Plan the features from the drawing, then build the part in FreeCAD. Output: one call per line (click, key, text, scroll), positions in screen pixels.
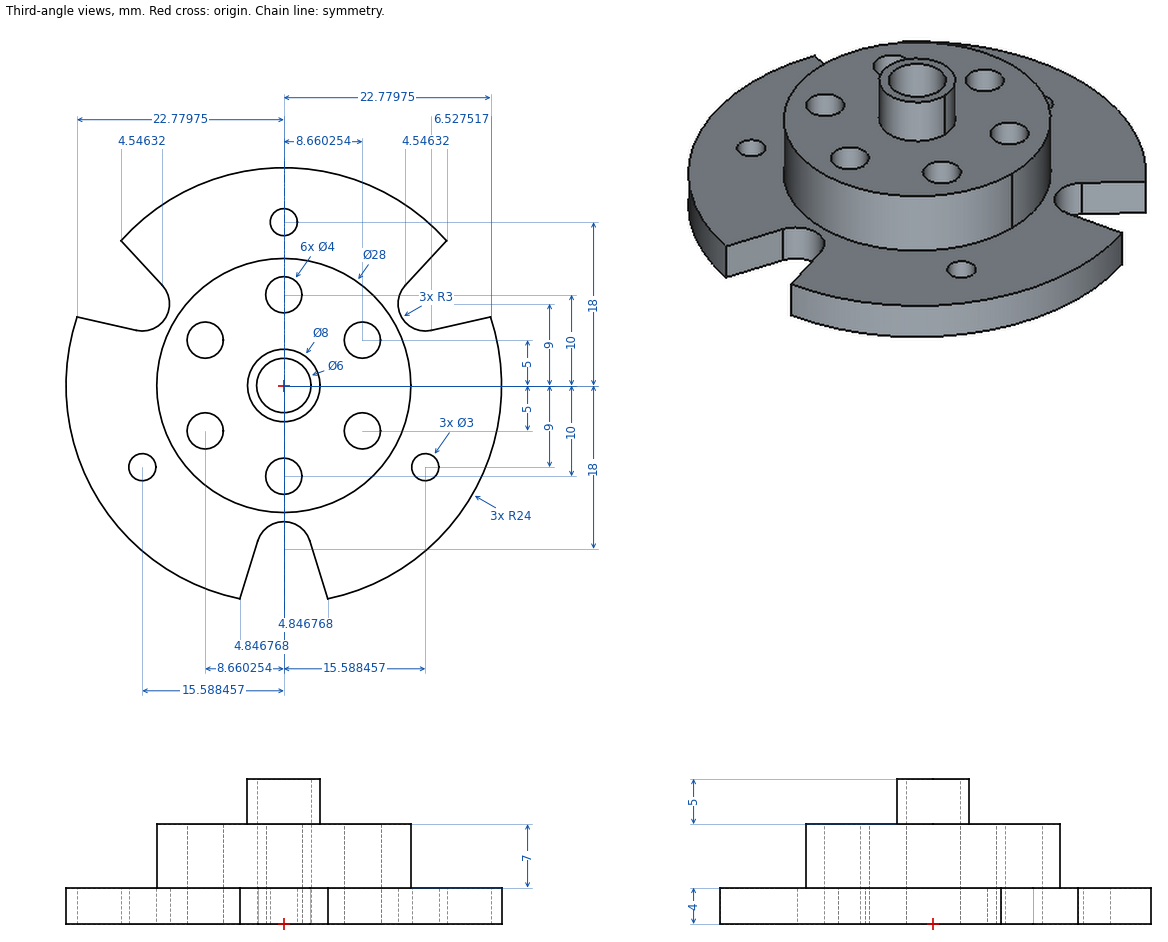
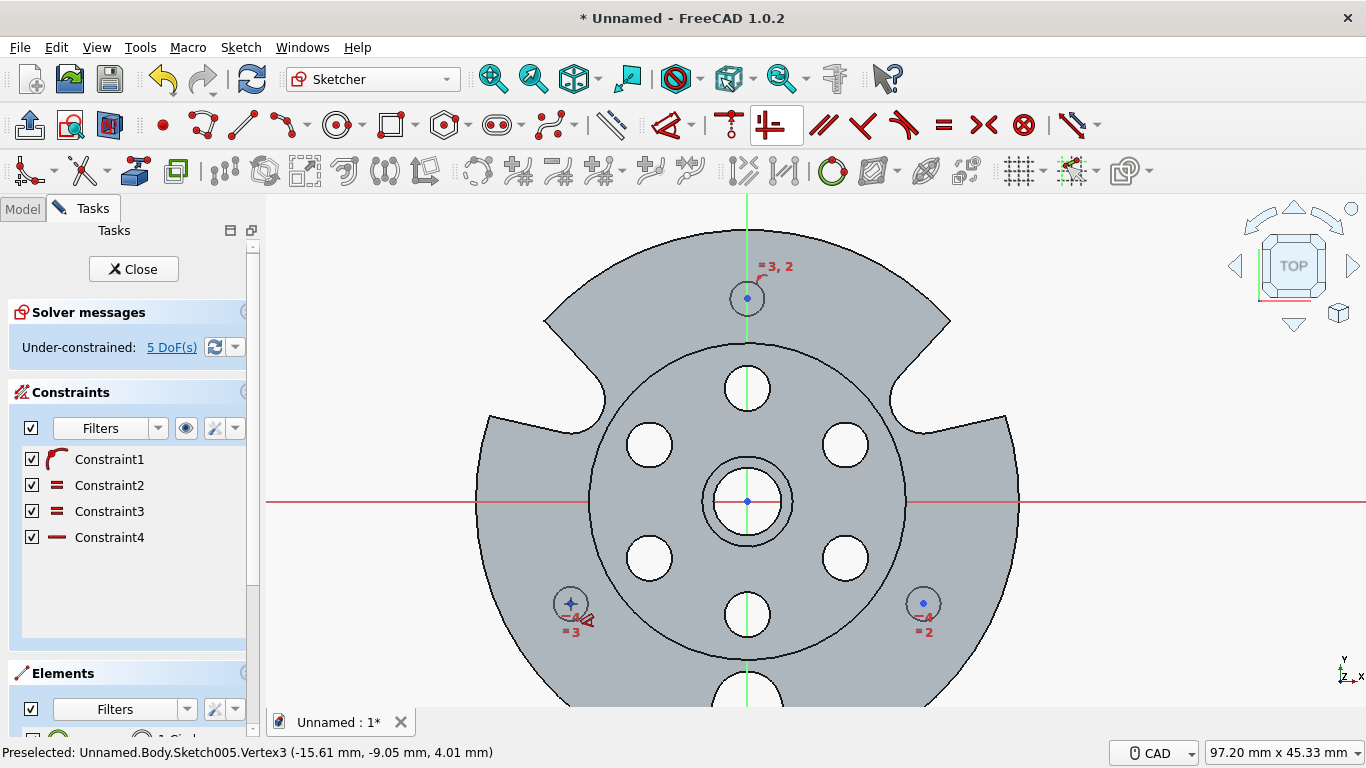
click(936, 592)
click(959, 570)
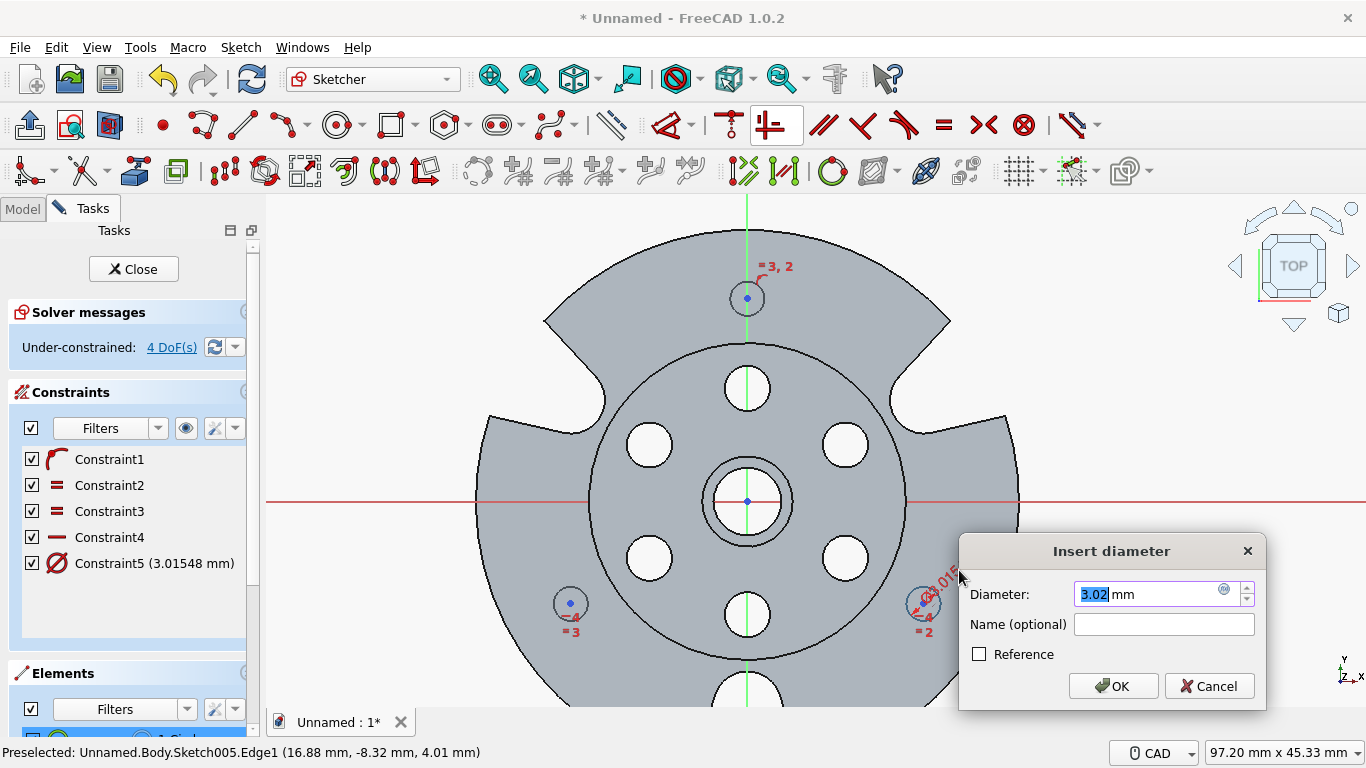
text(3)
key(Return)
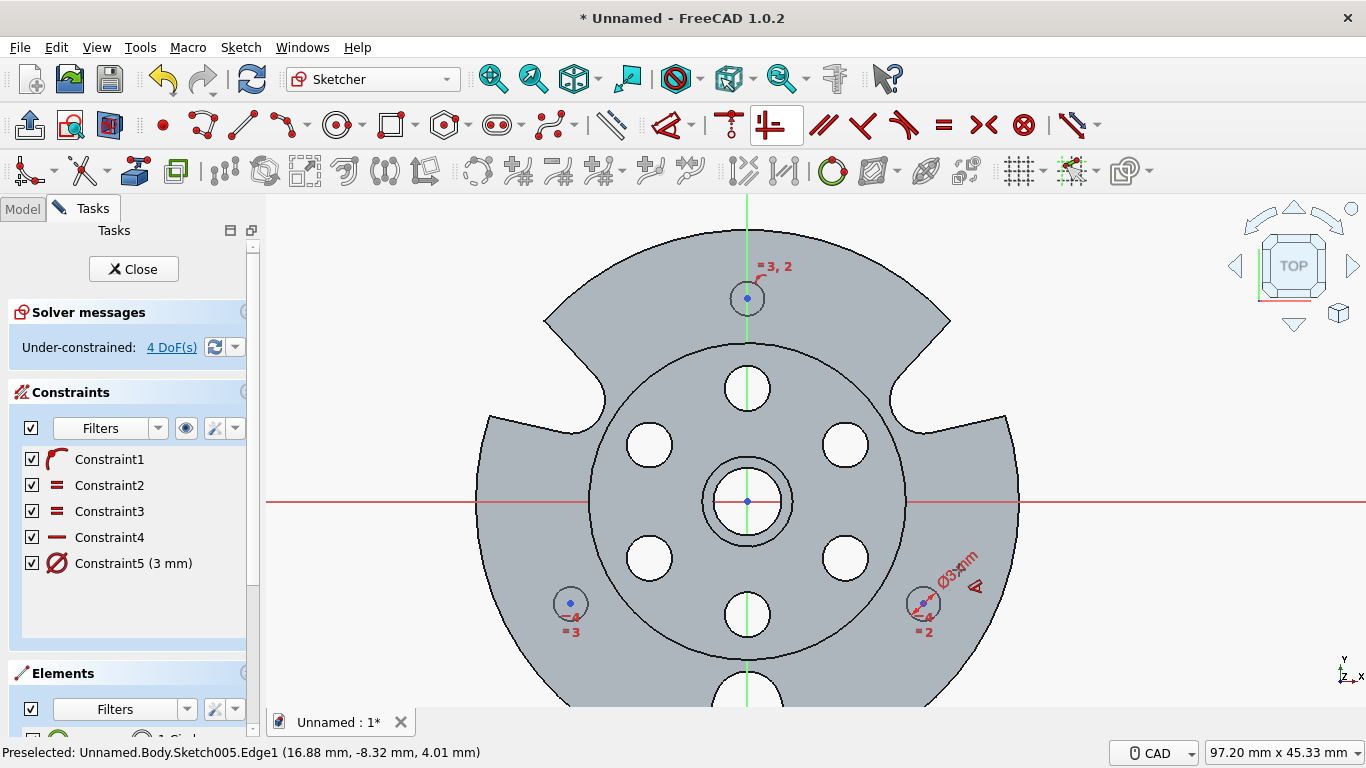
click(924, 604)
click(958, 529)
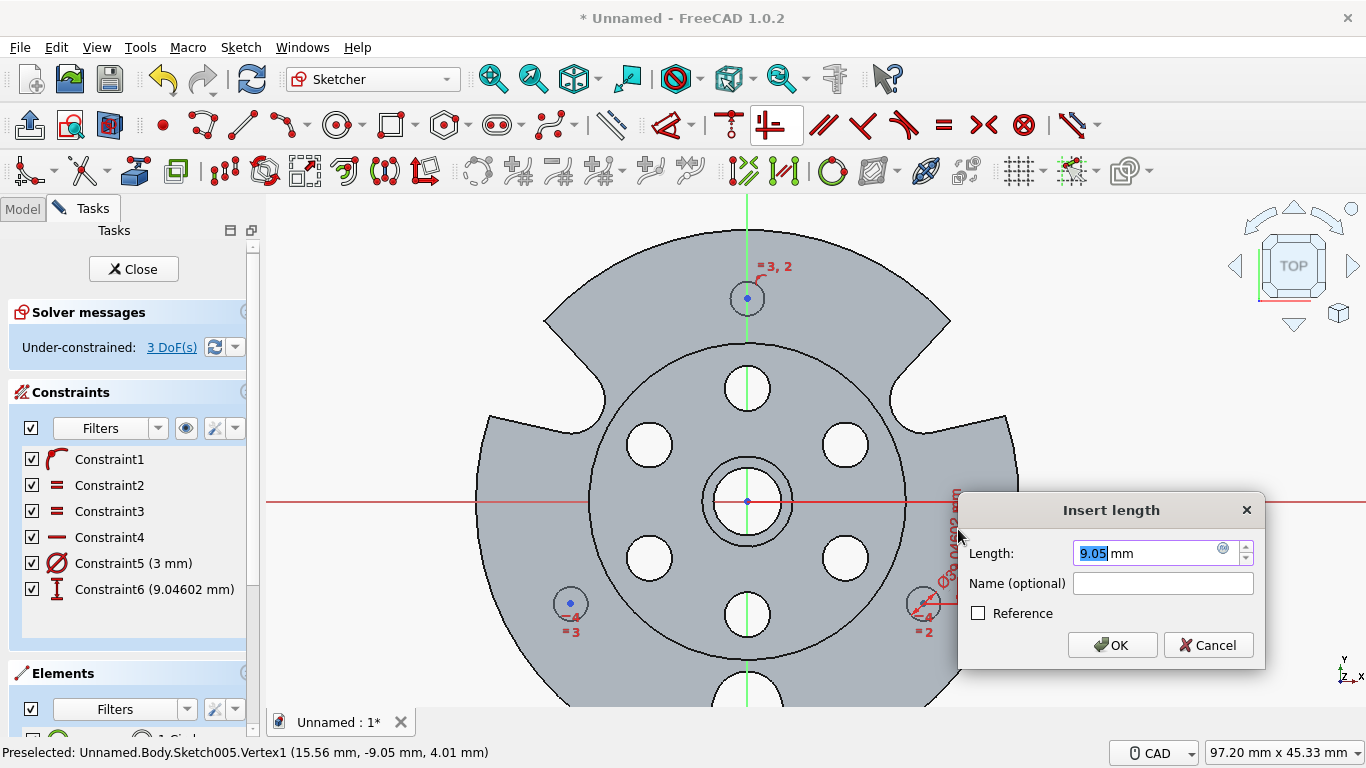
text(9)
key(Return)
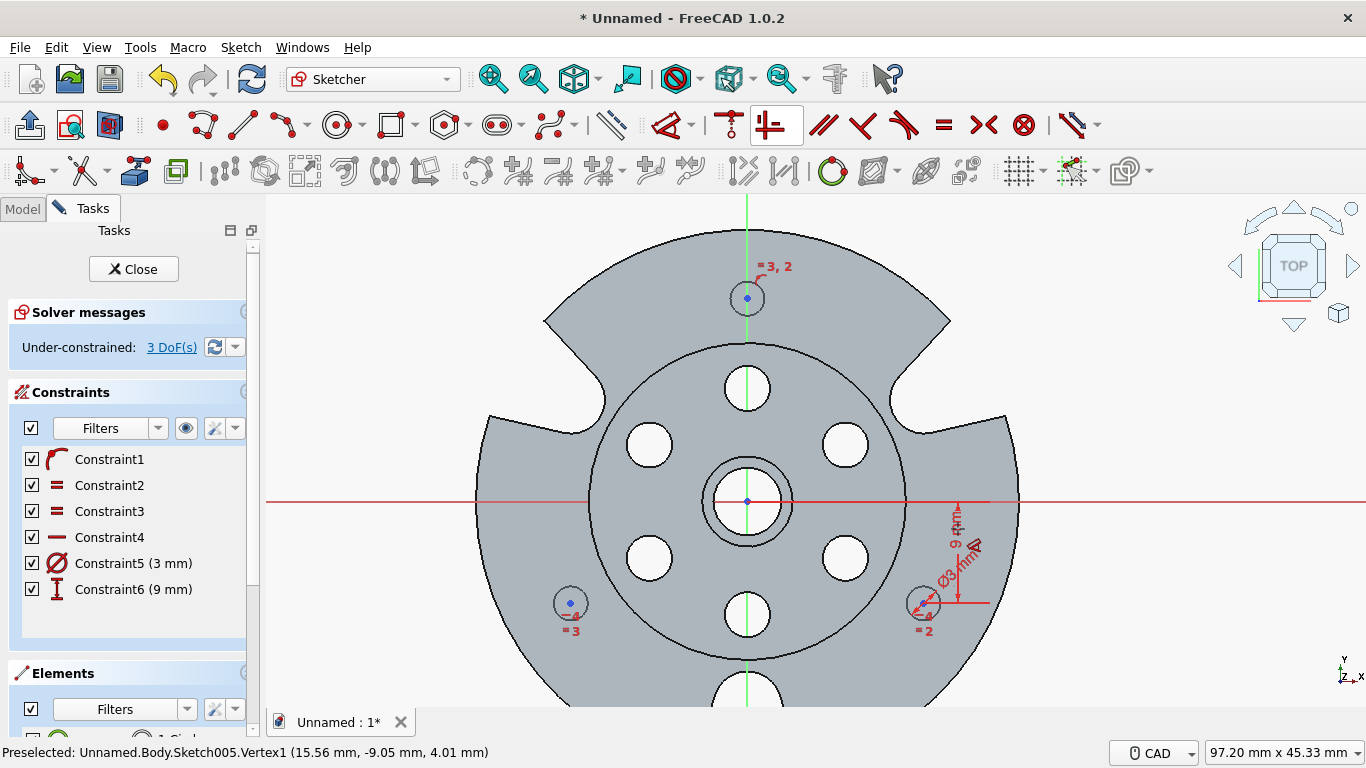
click(747, 299)
click(781, 400)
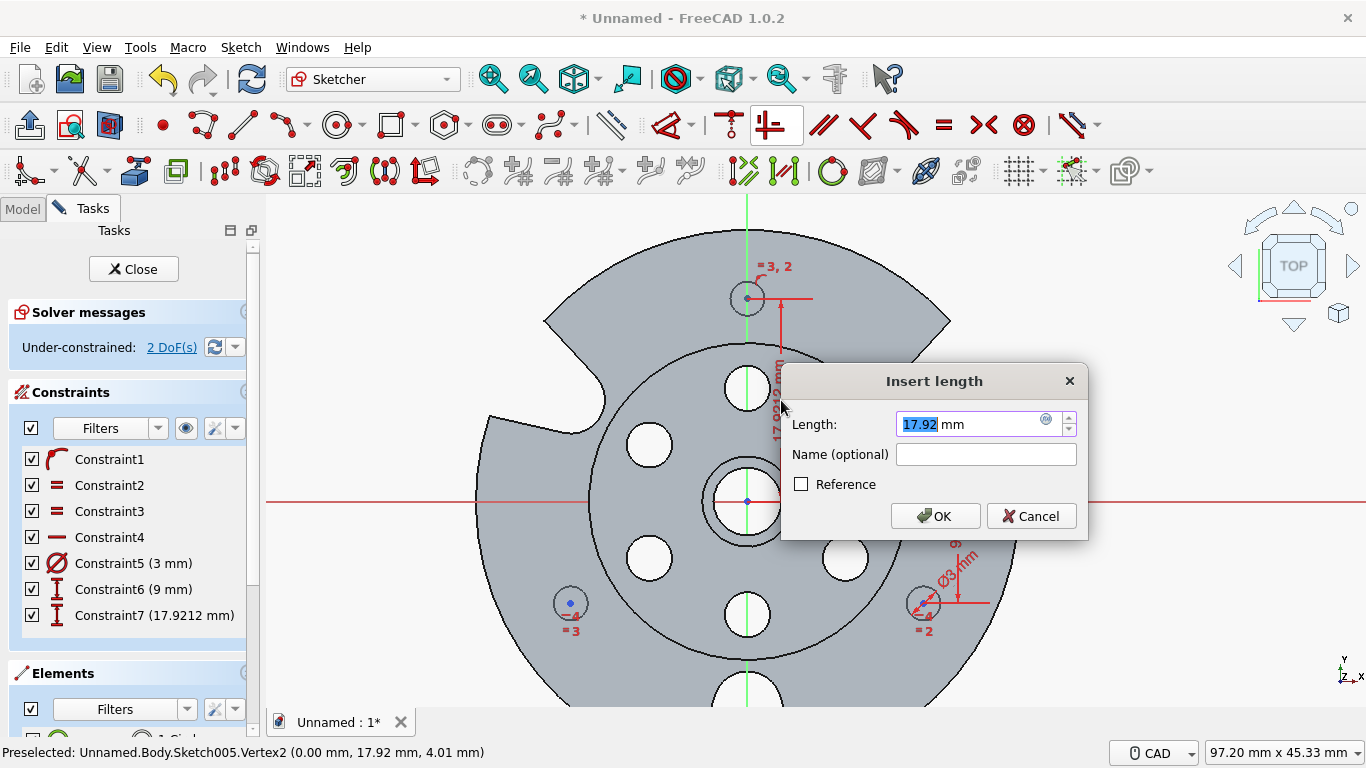
text(18)
key(Return)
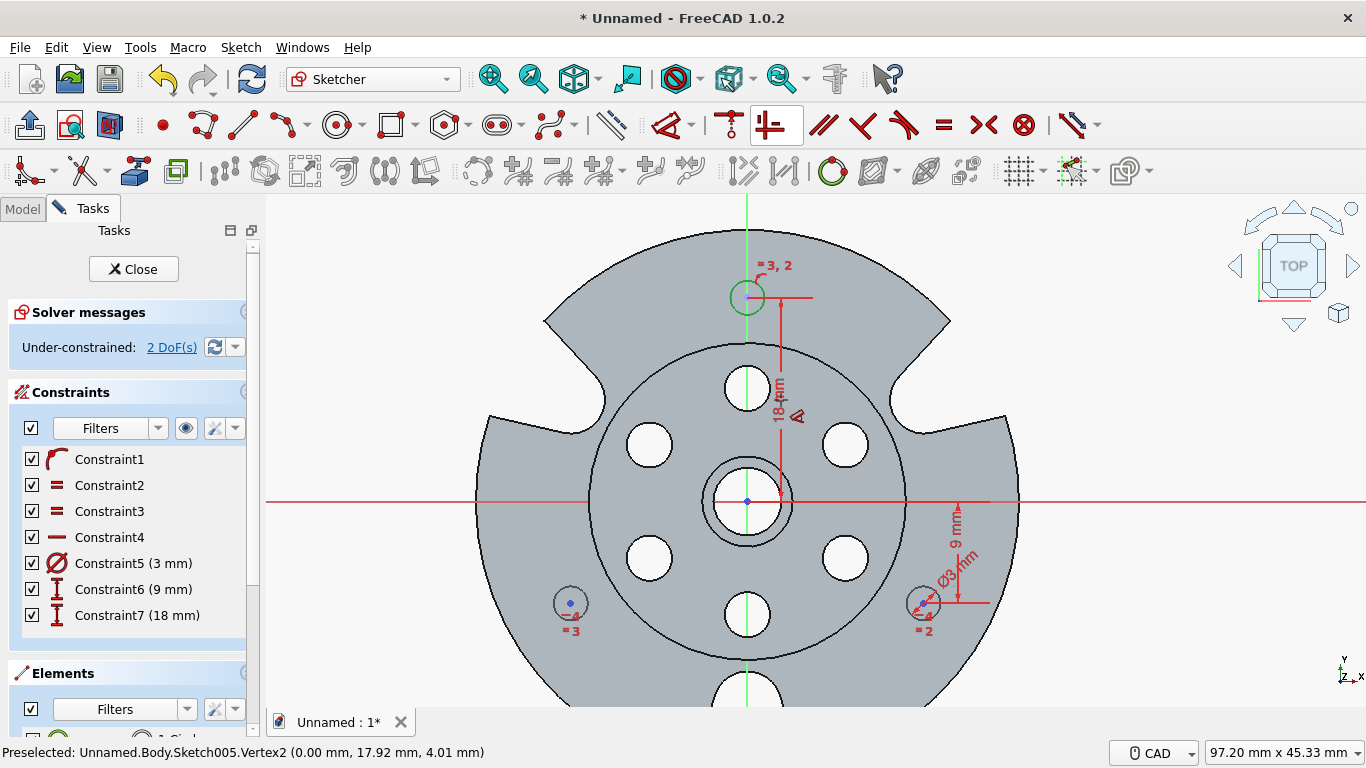
click(924, 603)
click(835, 637)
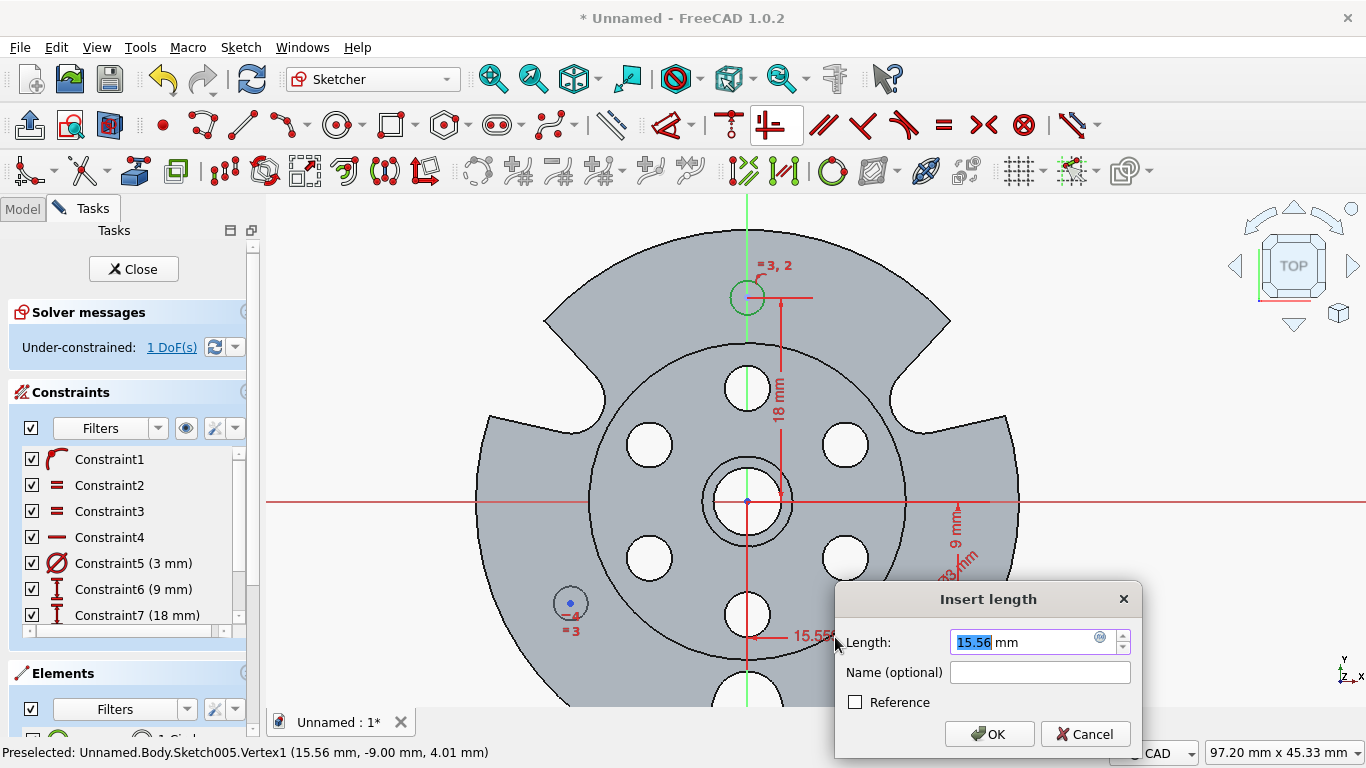
text(15.588457)
key(Return)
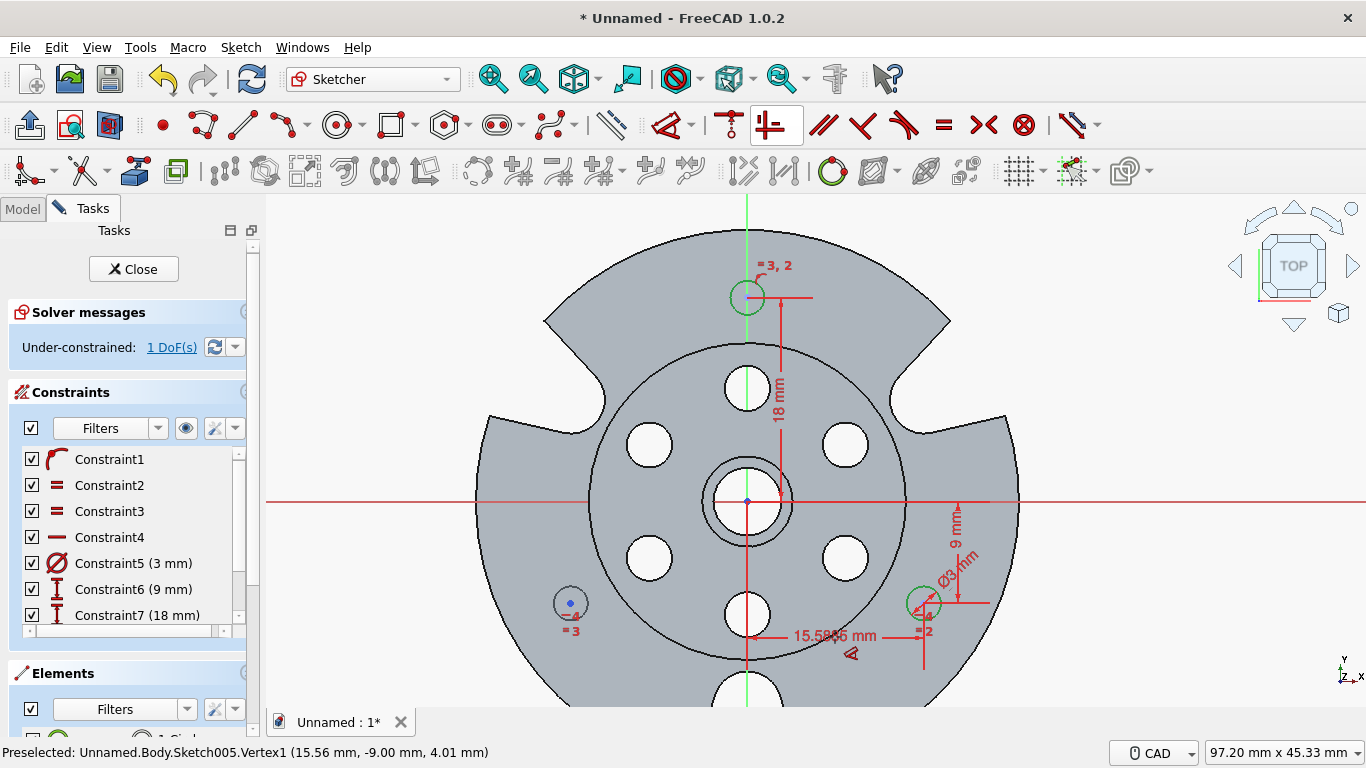
click(571, 603)
click(659, 637)